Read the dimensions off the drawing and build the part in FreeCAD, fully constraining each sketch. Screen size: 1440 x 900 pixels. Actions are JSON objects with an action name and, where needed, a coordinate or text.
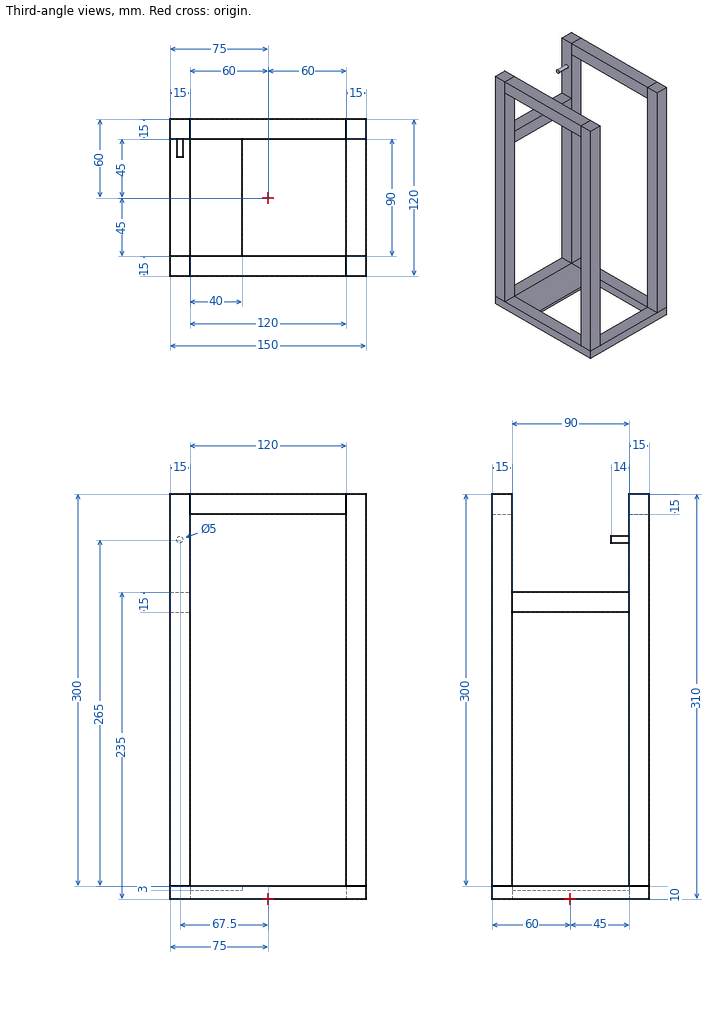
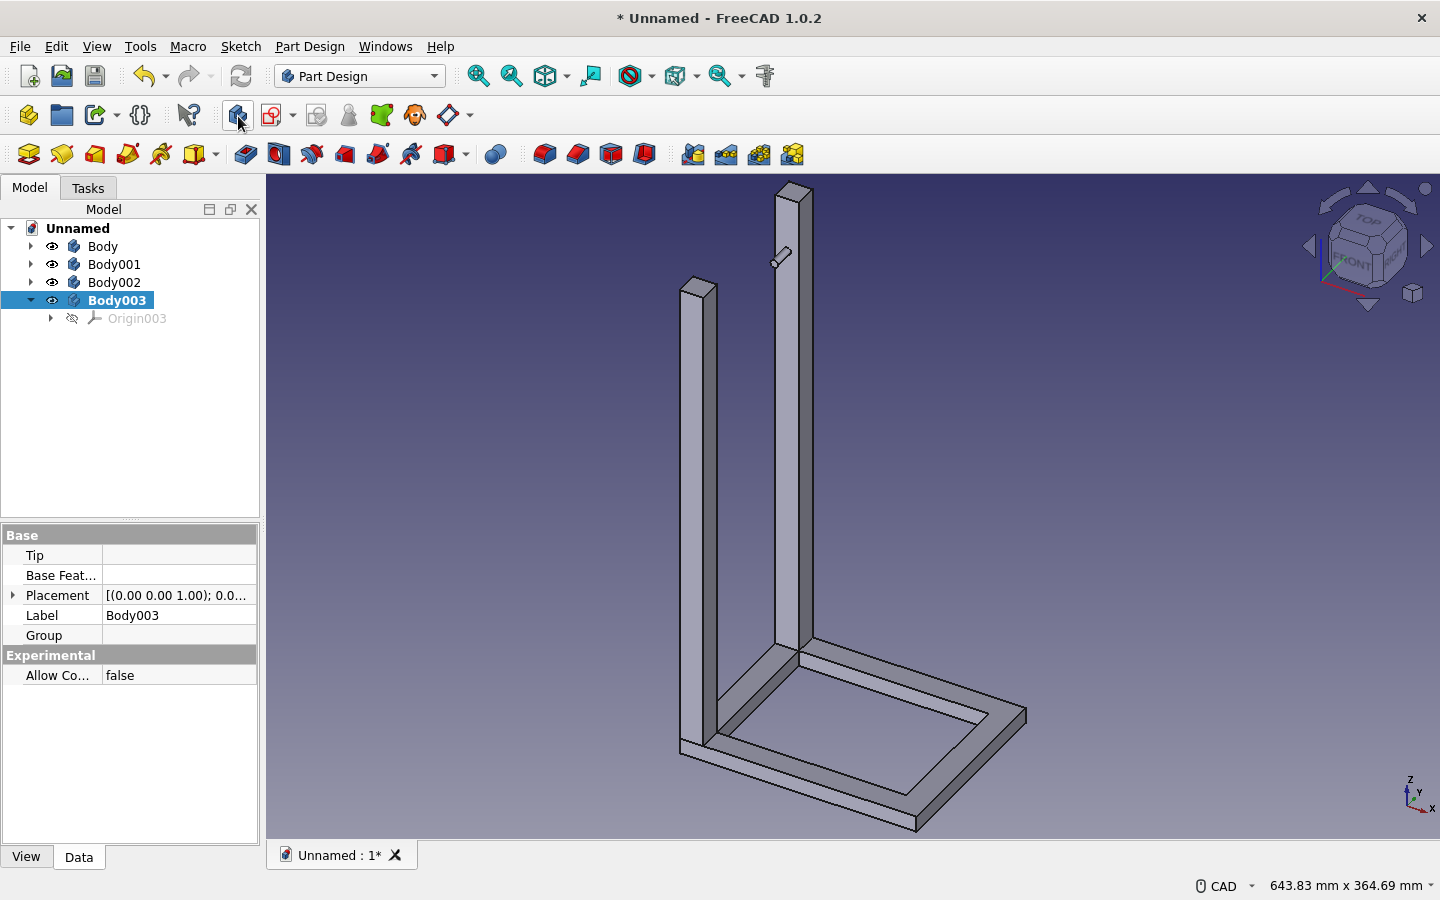
{"action": "left_click", "coordinate": [51, 318]}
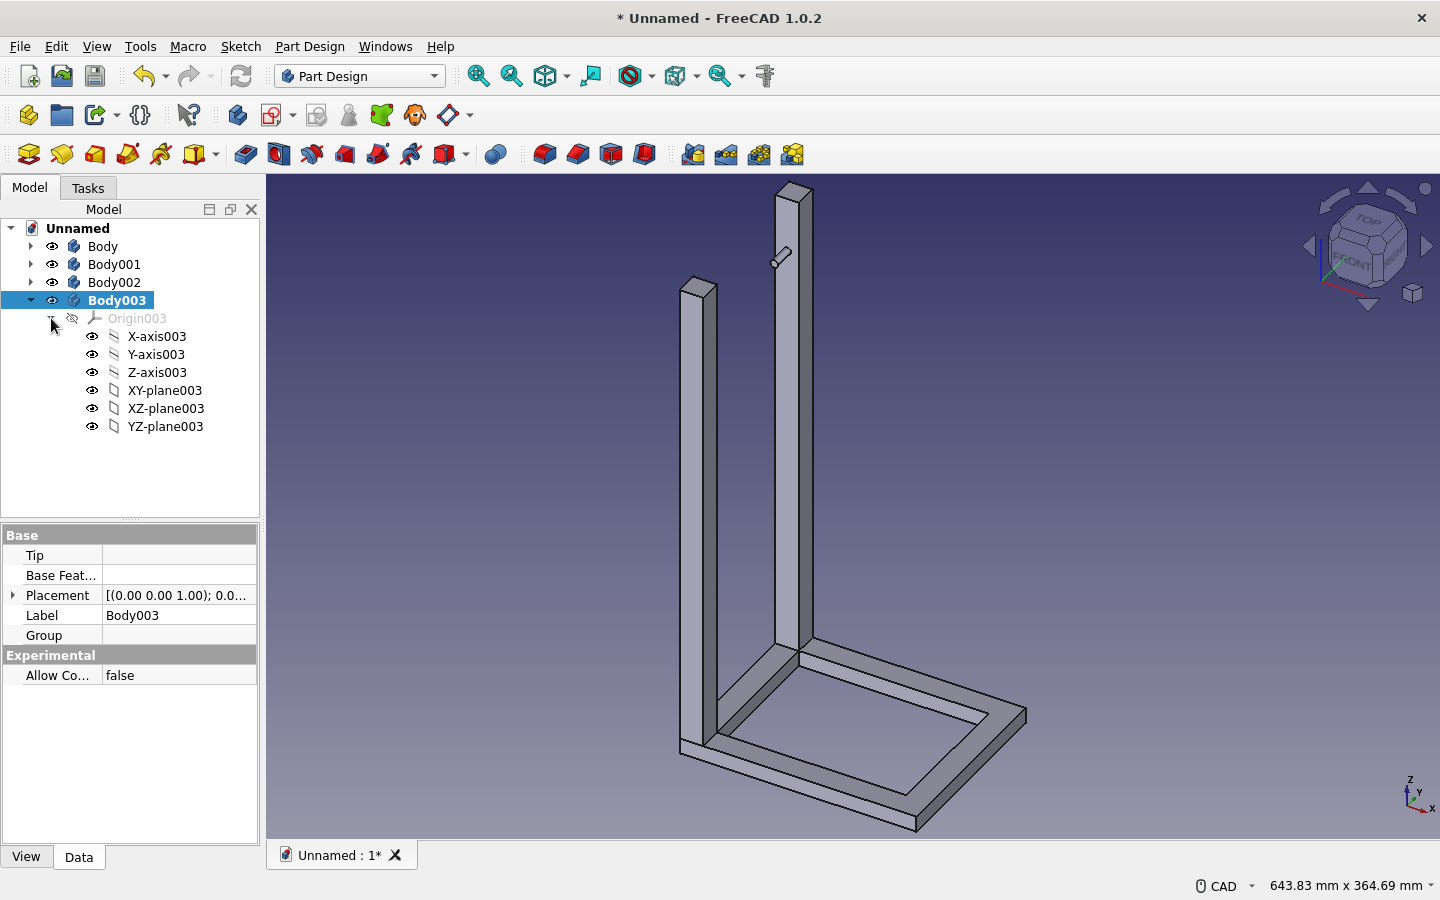
{"action": "left_click", "coordinate": [137, 390]}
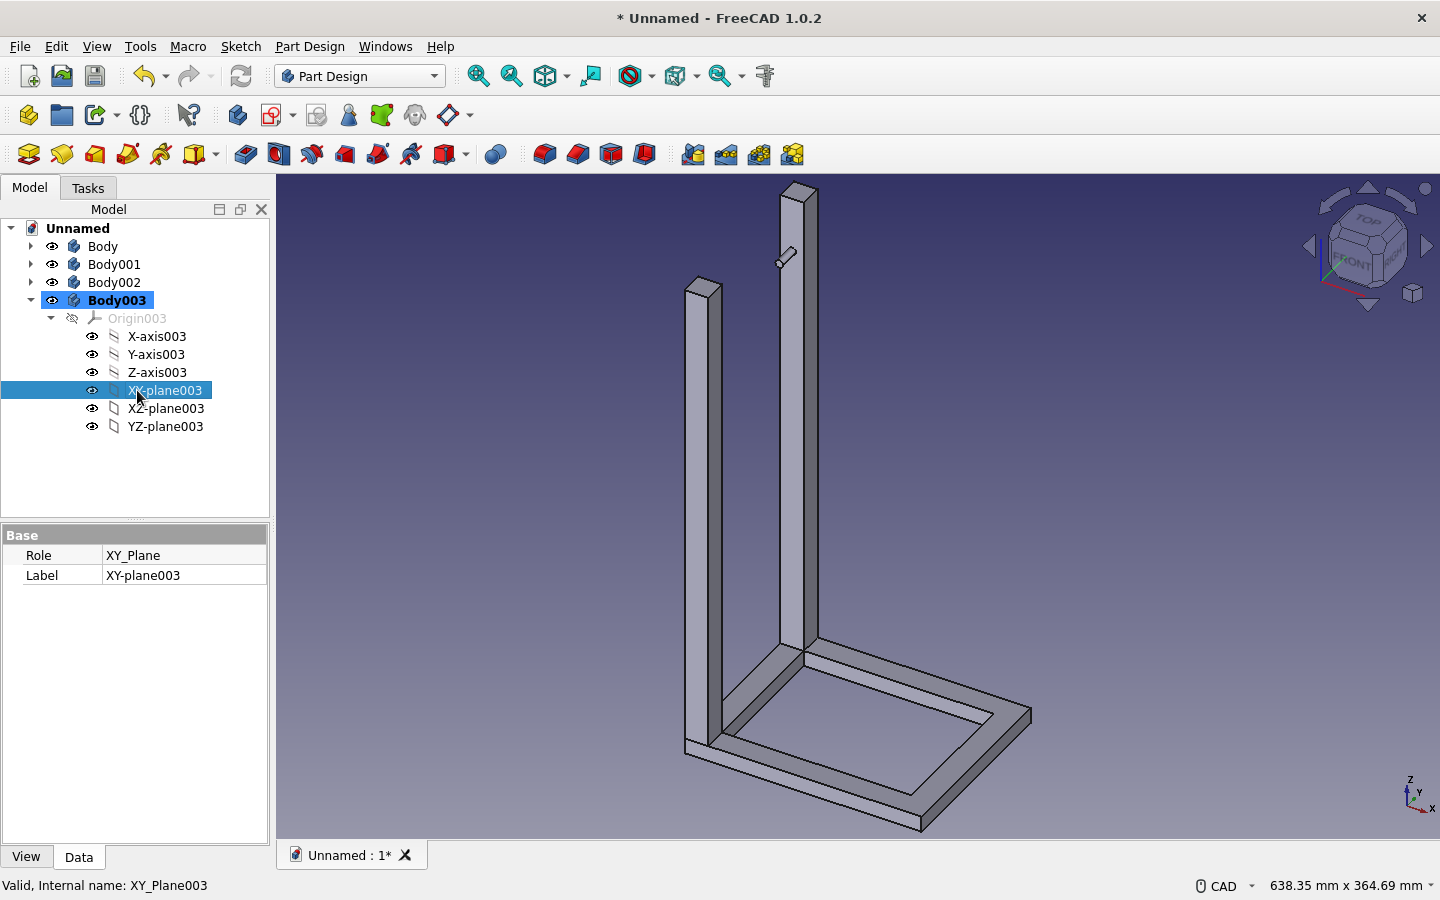
{"action": "left_click", "coordinate": [448, 116]}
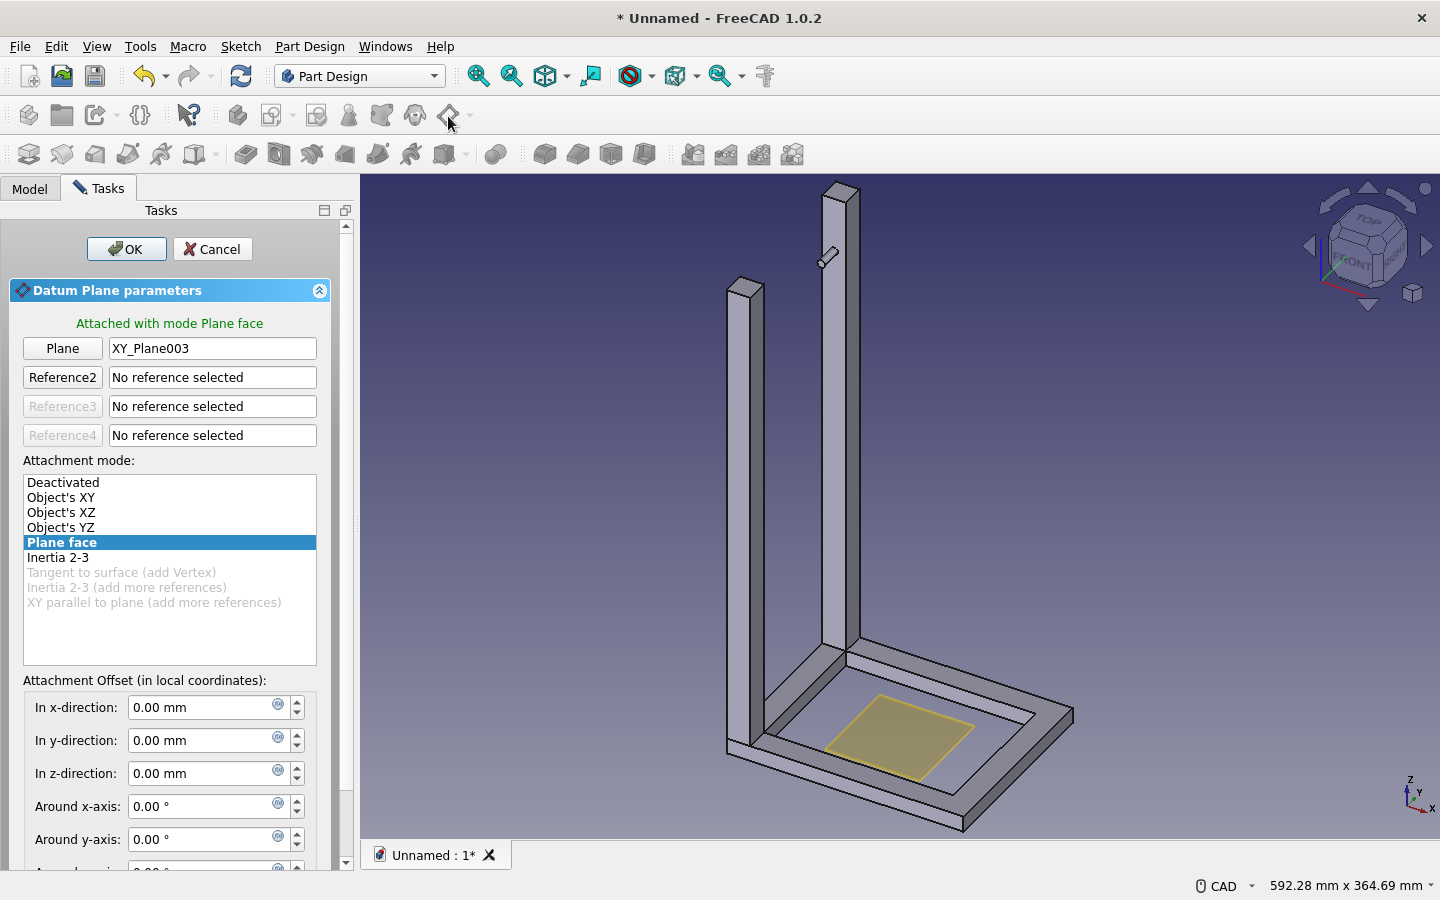
{"action": "triple_click", "coordinate": [210, 774]}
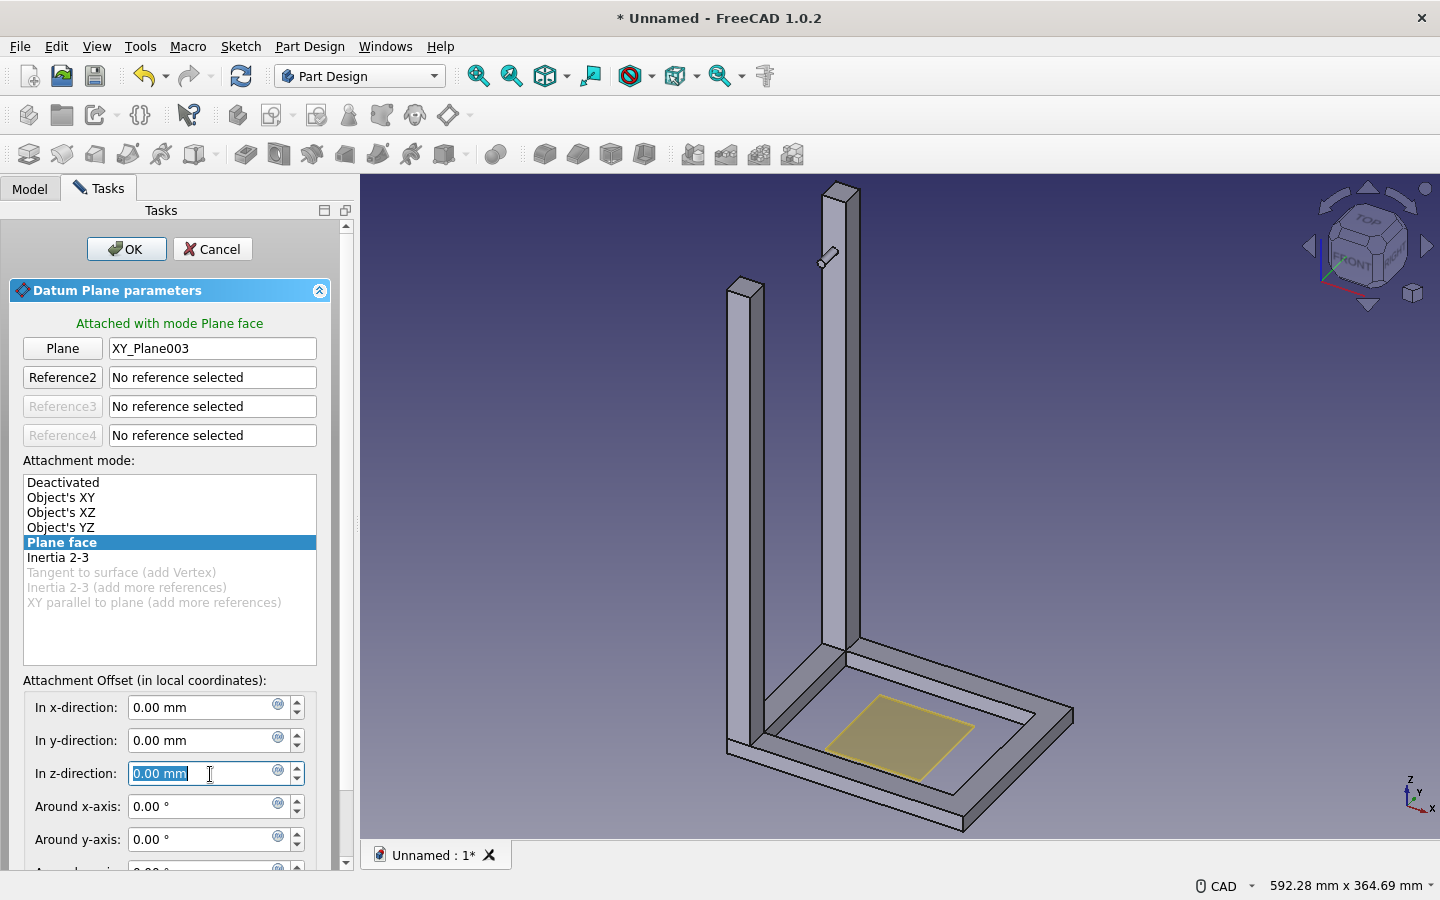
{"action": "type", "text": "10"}
{"action": "key", "text": "Tab"}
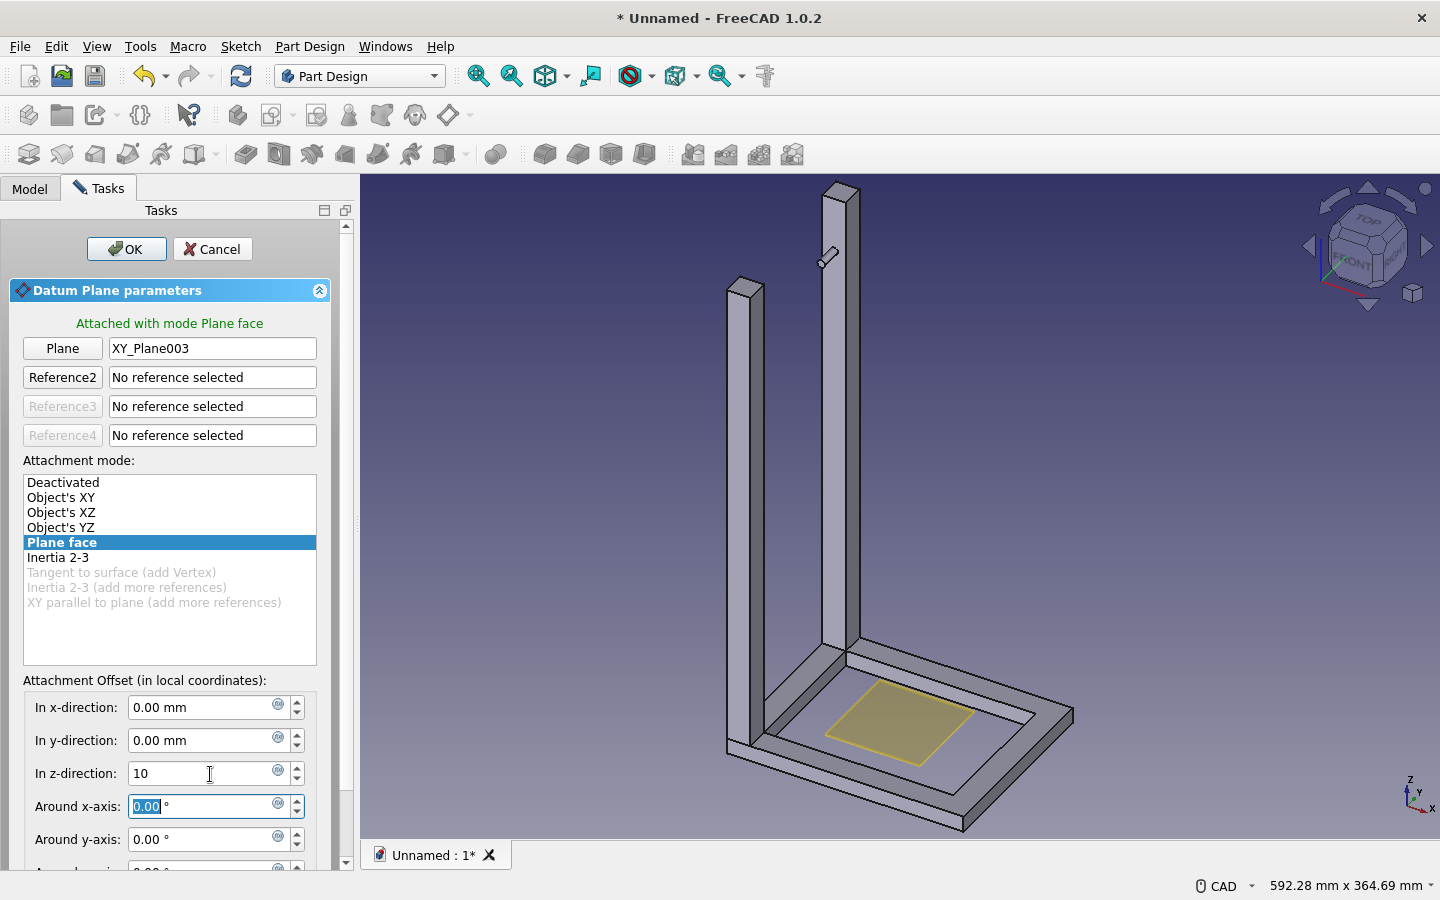
{"action": "left_click", "coordinate": [127, 249]}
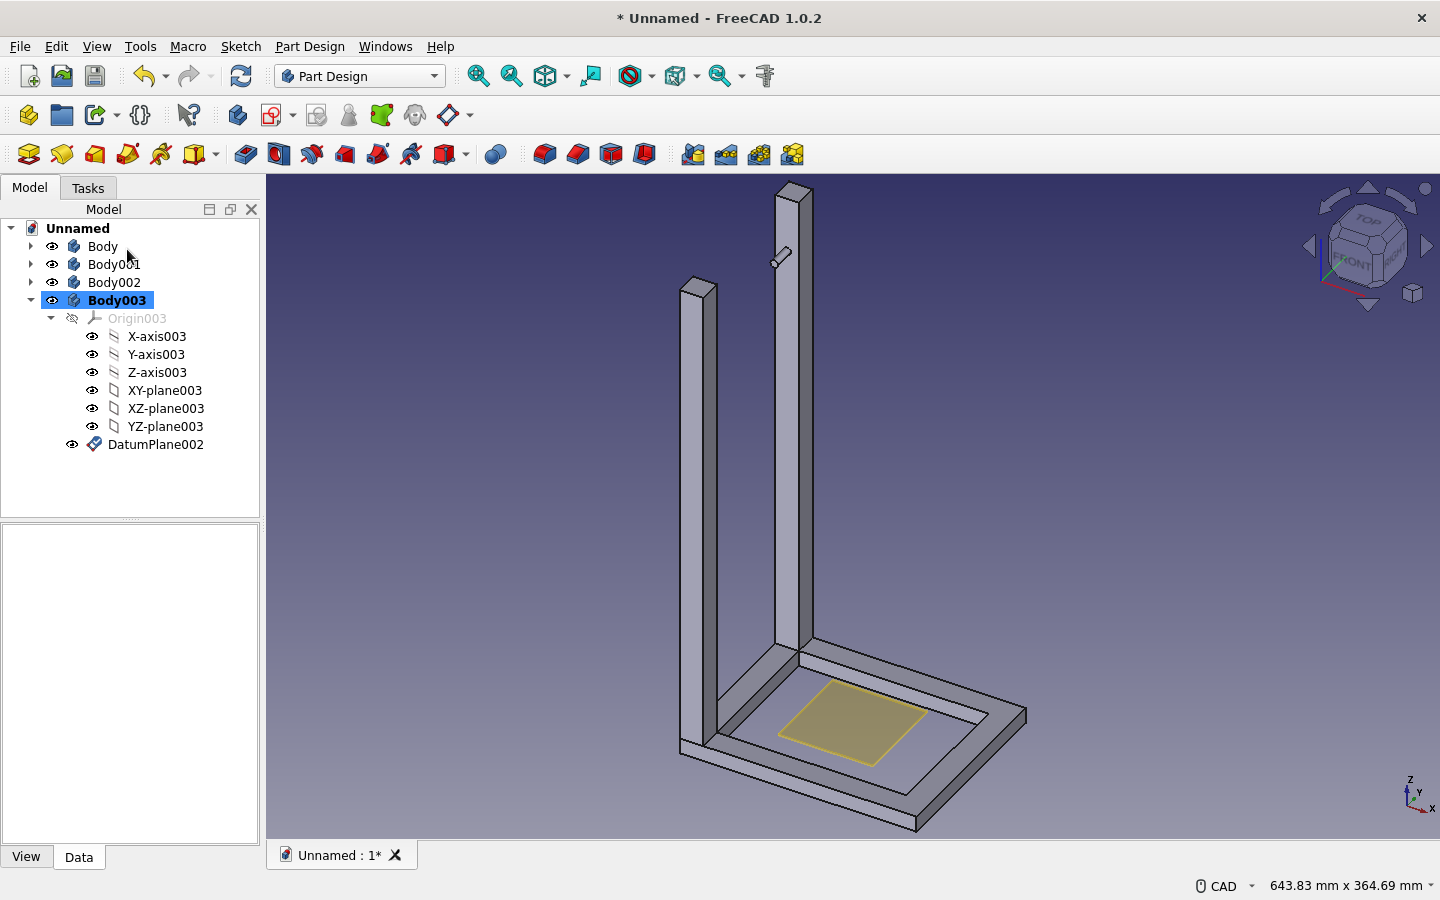
{"action": "left_click", "coordinate": [117, 444]}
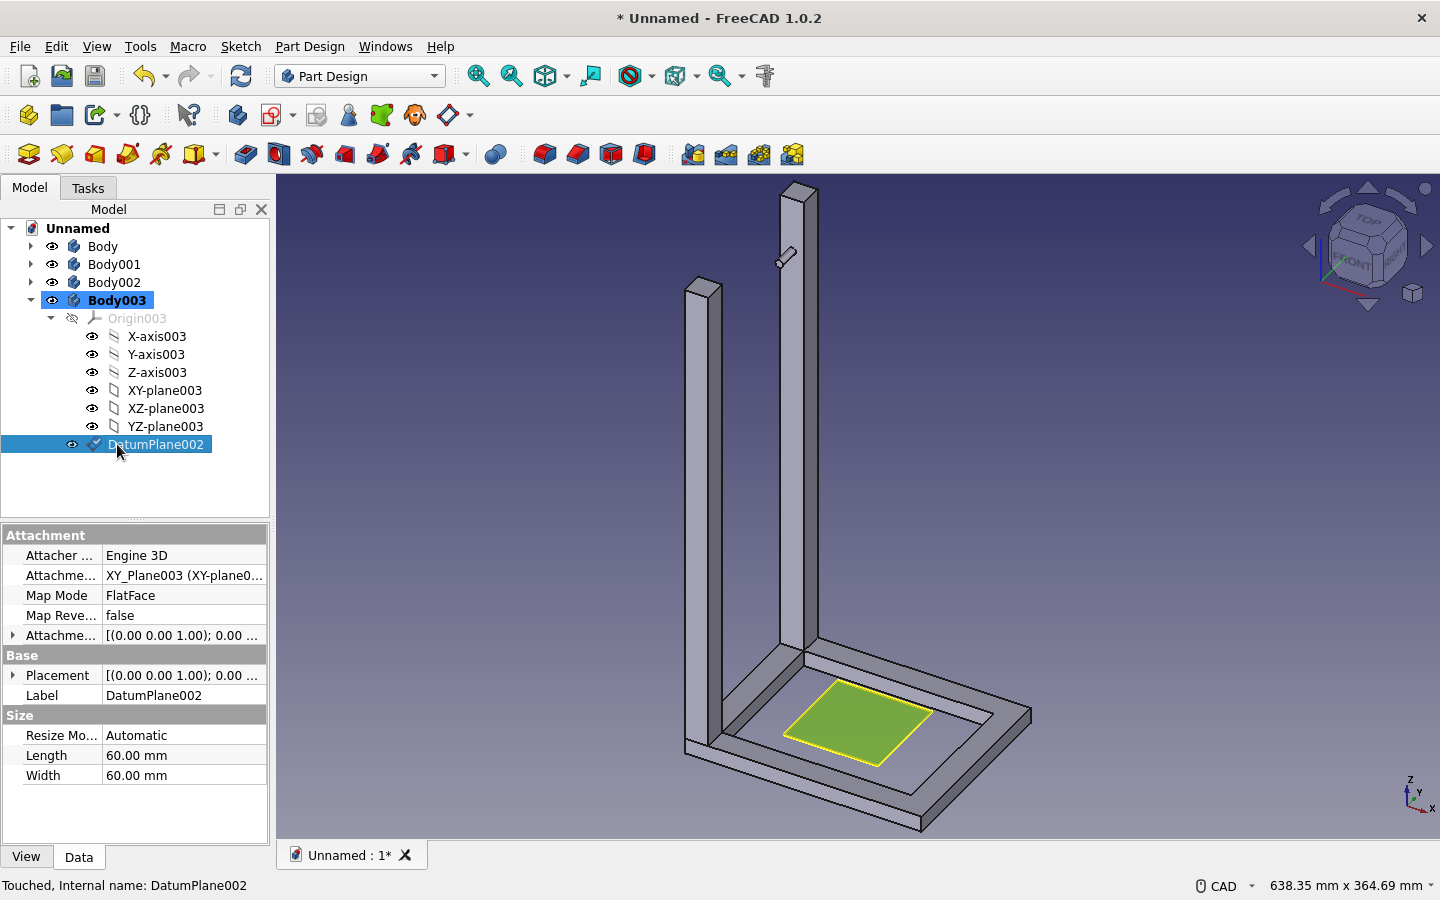
{"action": "left_click", "coordinate": [270, 116]}